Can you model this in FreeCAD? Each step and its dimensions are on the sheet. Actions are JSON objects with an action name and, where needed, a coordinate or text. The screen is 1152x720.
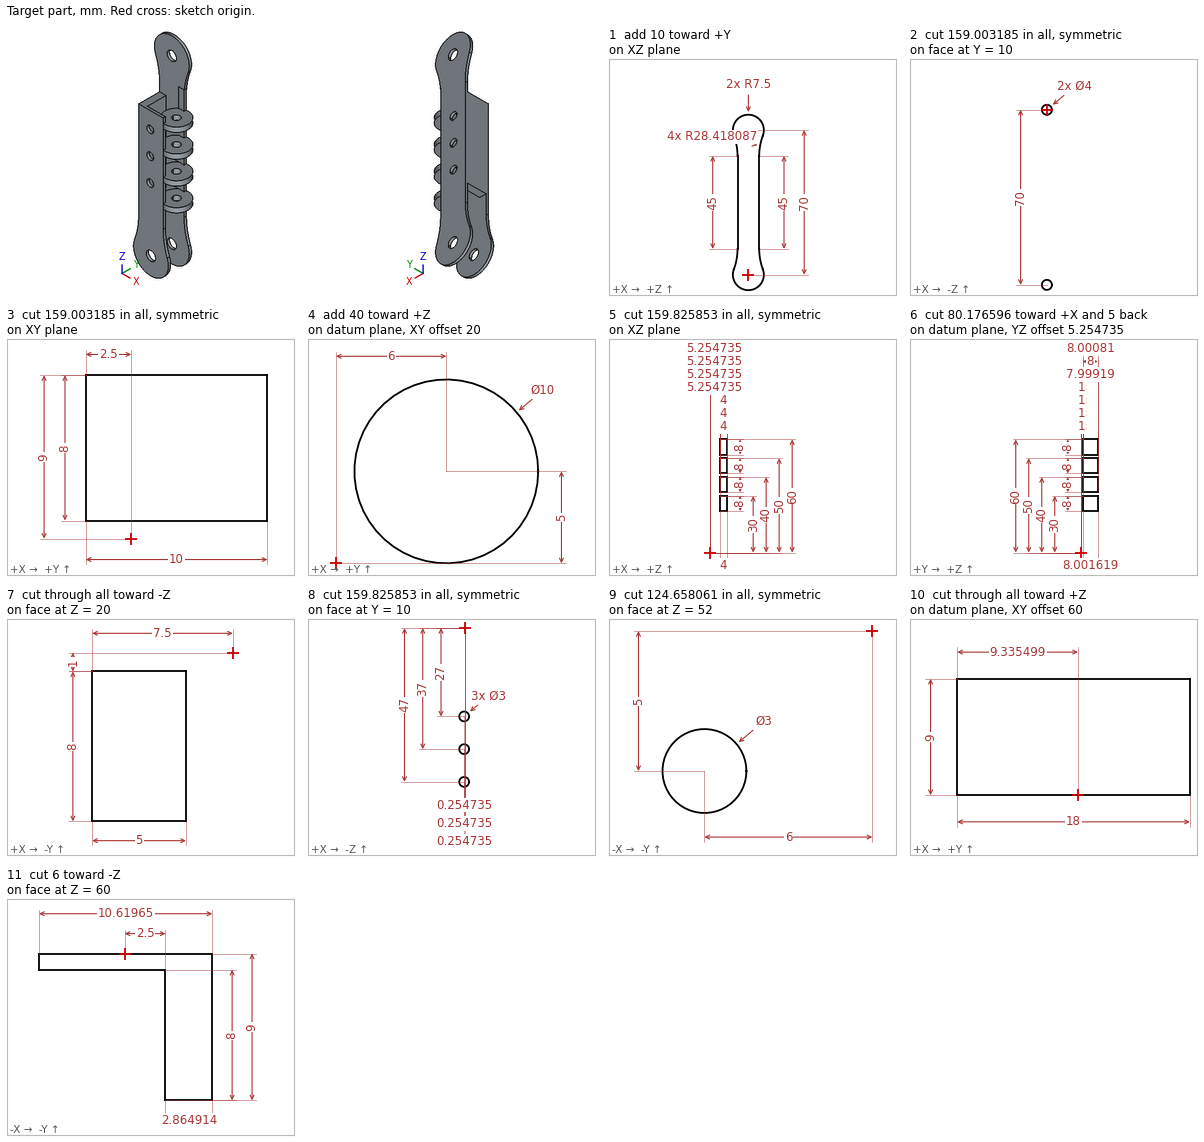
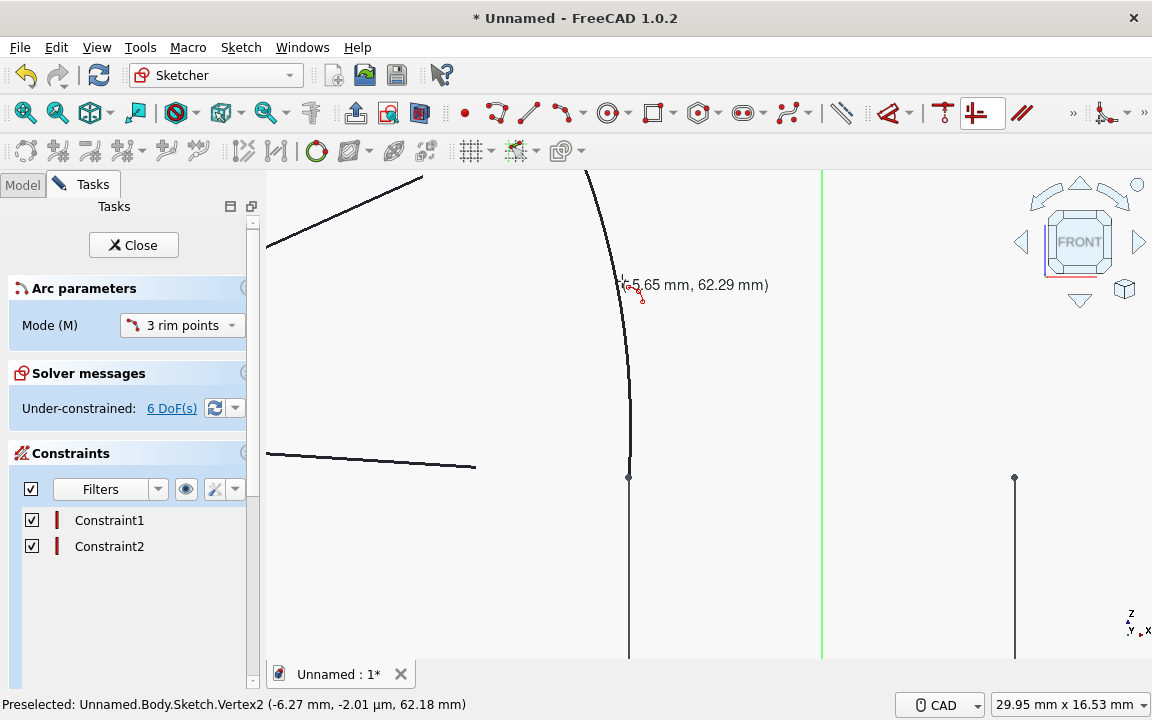
{"action": "left_click", "coordinate": [616, 281]}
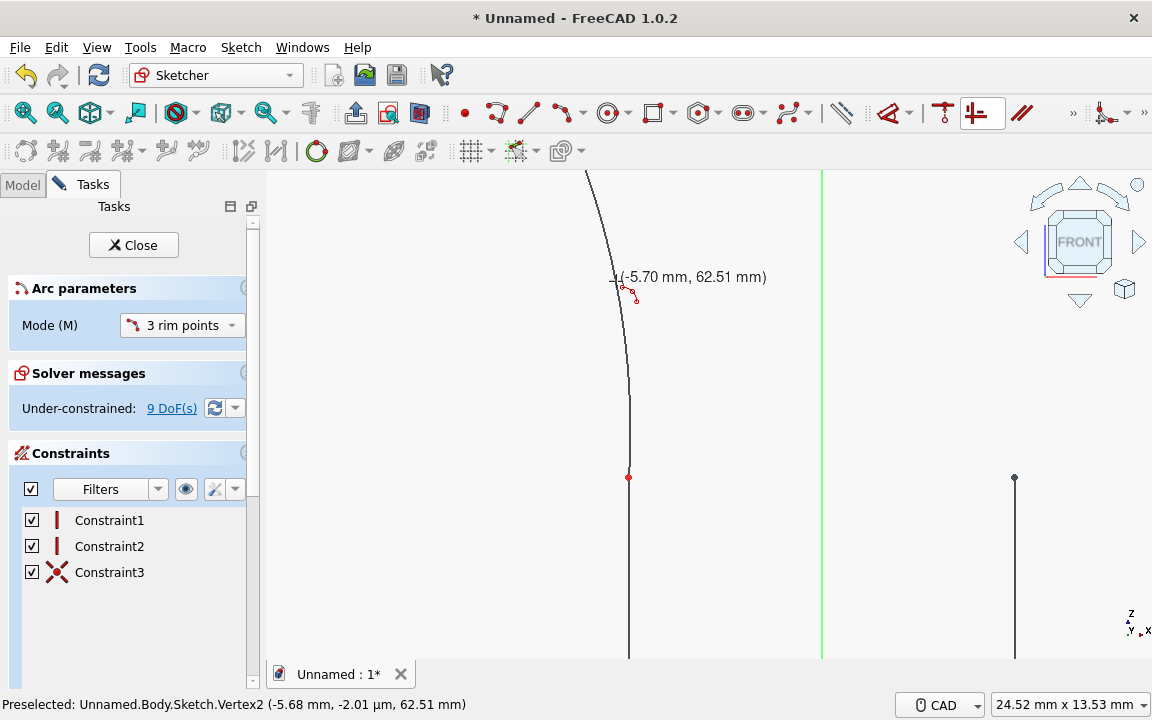
{"action": "scroll", "coordinate": [622, 329], "scroll_direction": "down", "scroll_amount": 12}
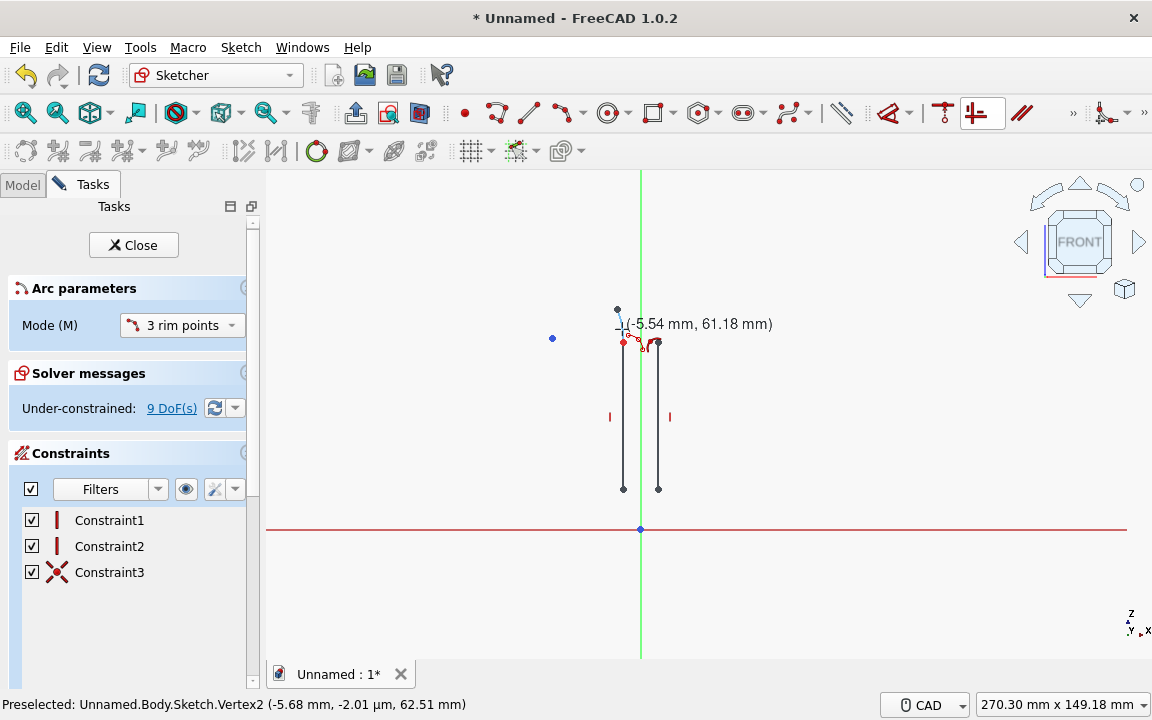
{"action": "left_click", "coordinate": [617, 310]}
{"action": "left_click", "coordinate": [664, 309]}
{"action": "left_click", "coordinate": [658, 283]}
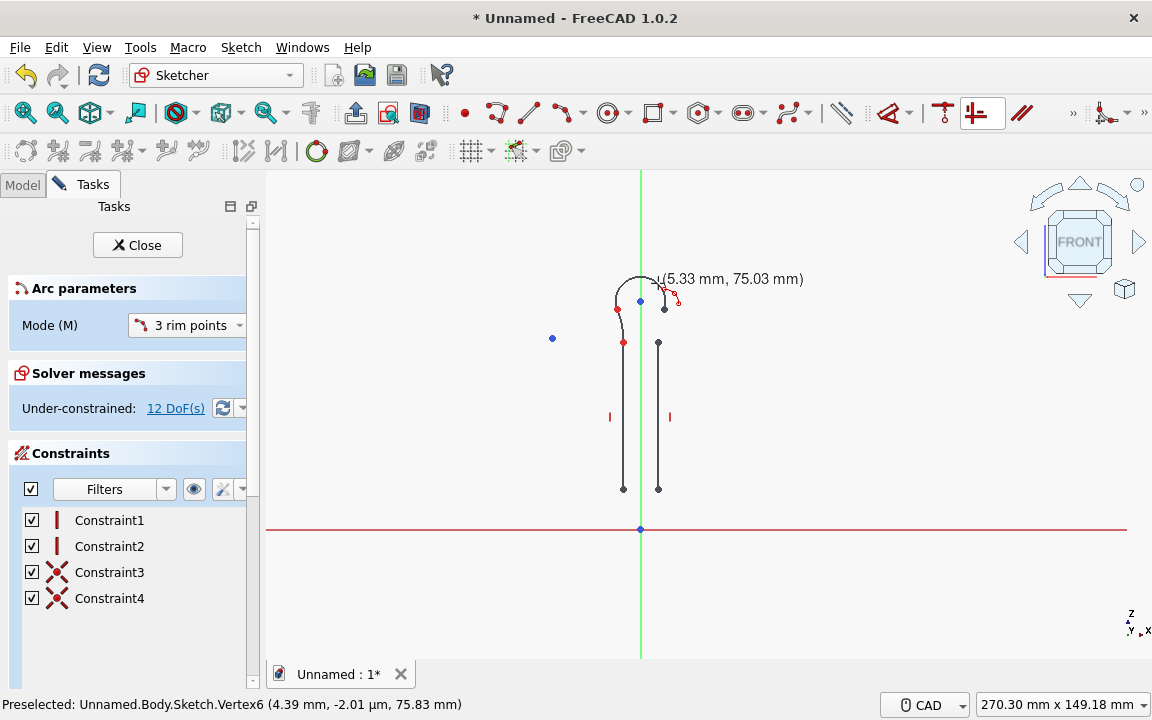
{"action": "left_click", "coordinate": [664, 310]}
{"action": "left_click", "coordinate": [658, 343]}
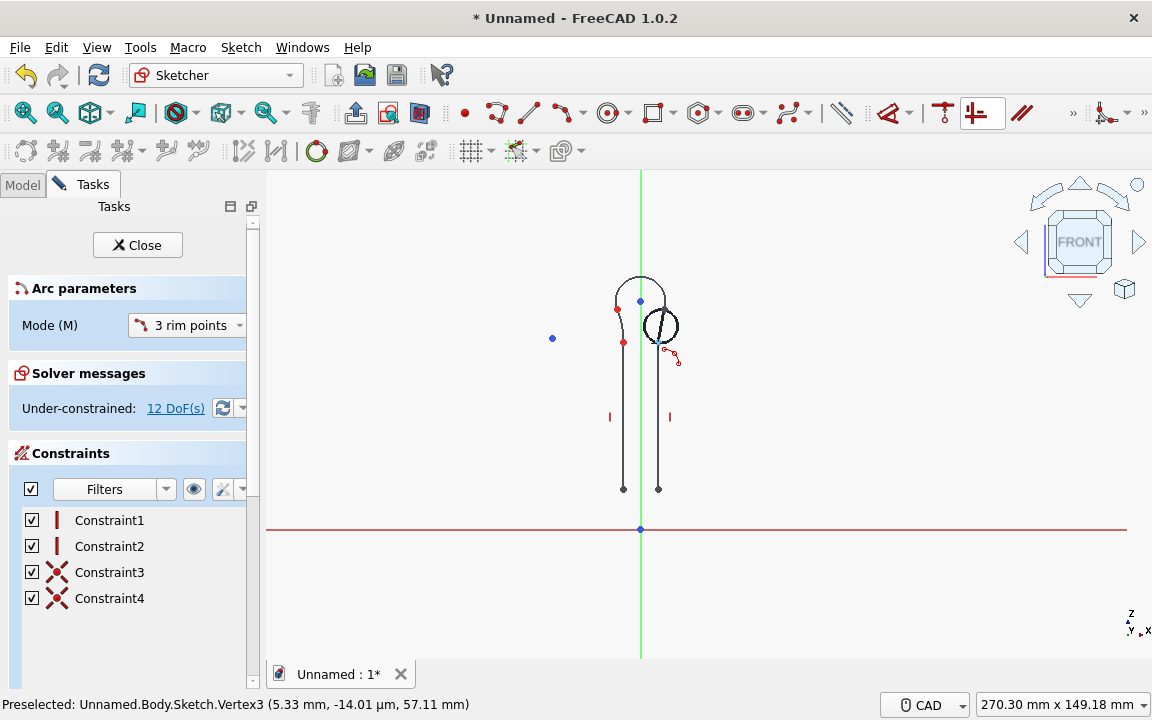
{"action": "scroll", "coordinate": [659, 325], "scroll_direction": "up", "scroll_amount": 12}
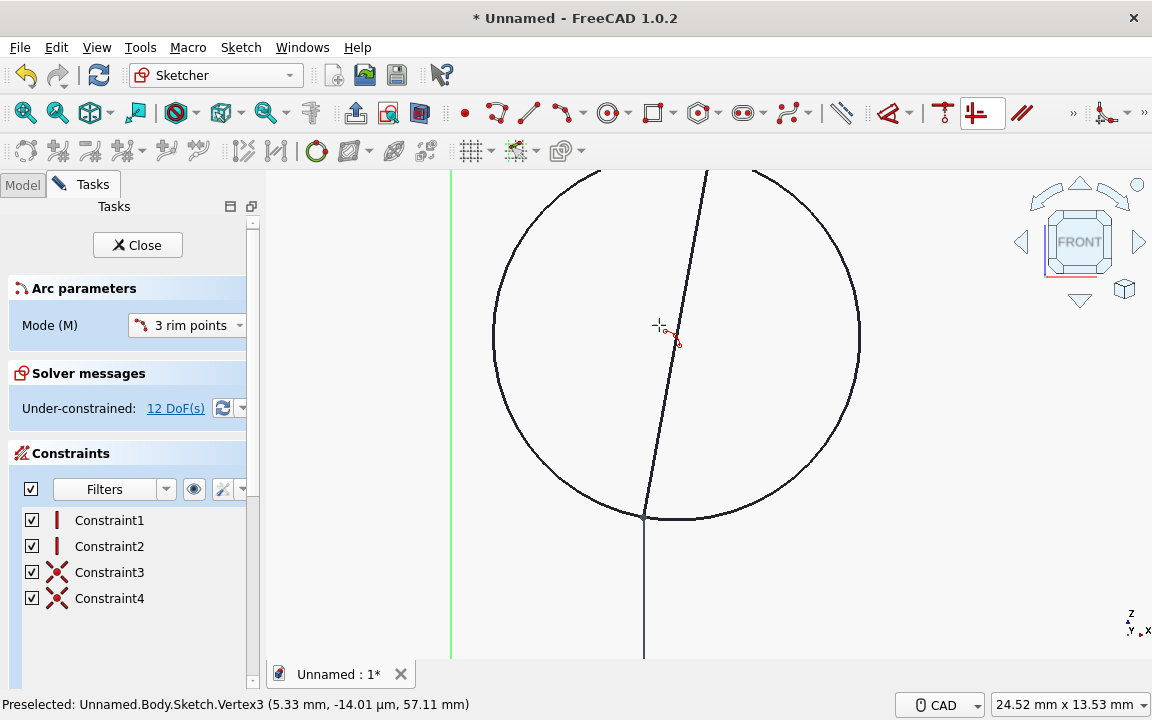
{"action": "left_click", "coordinate": [657, 322]}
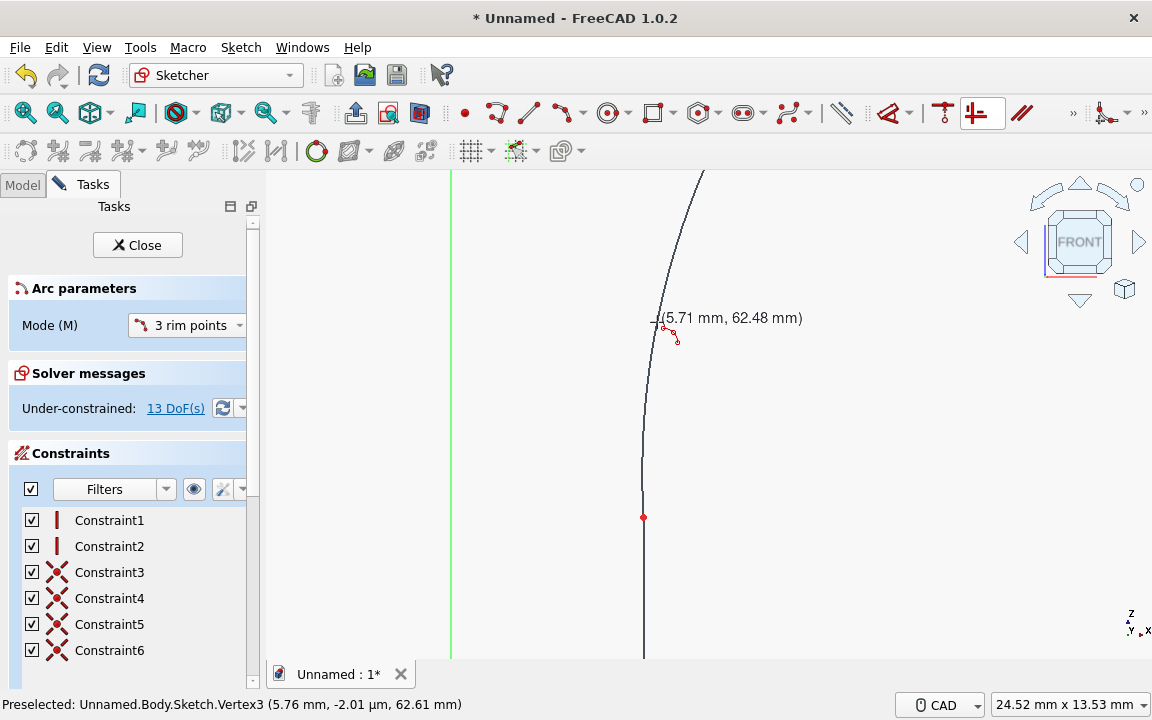
{"action": "scroll", "coordinate": [659, 325], "scroll_direction": "down", "scroll_amount": 12}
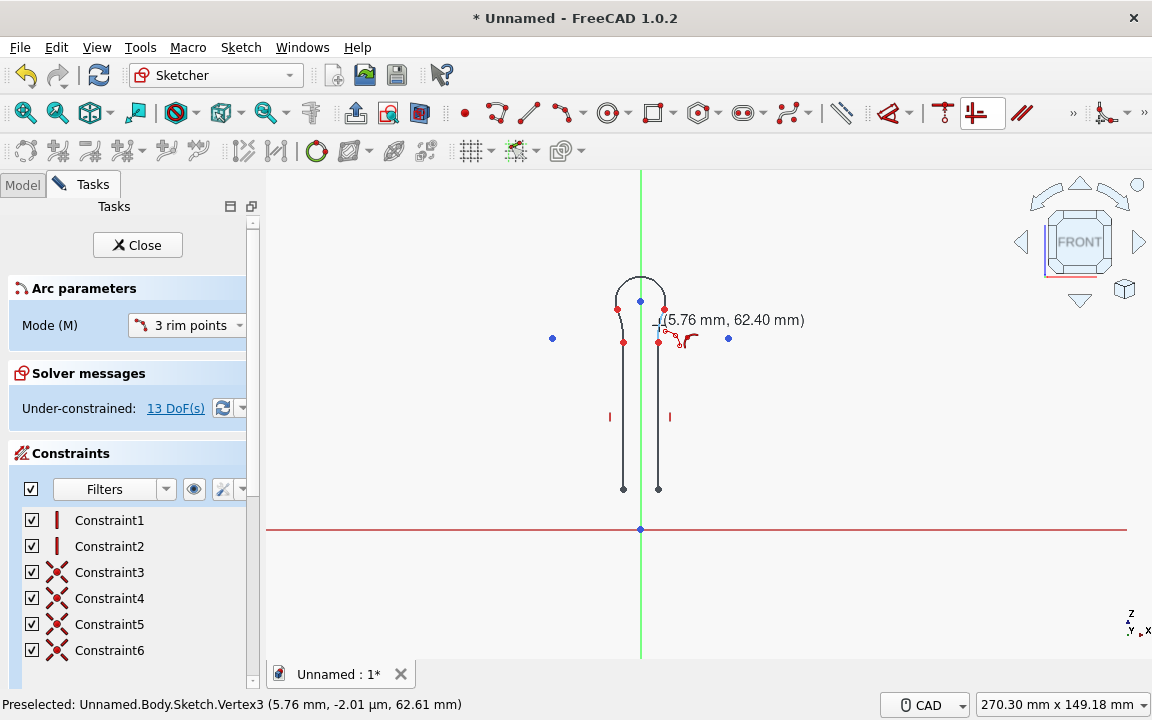
{"action": "left_click", "coordinate": [658, 490]}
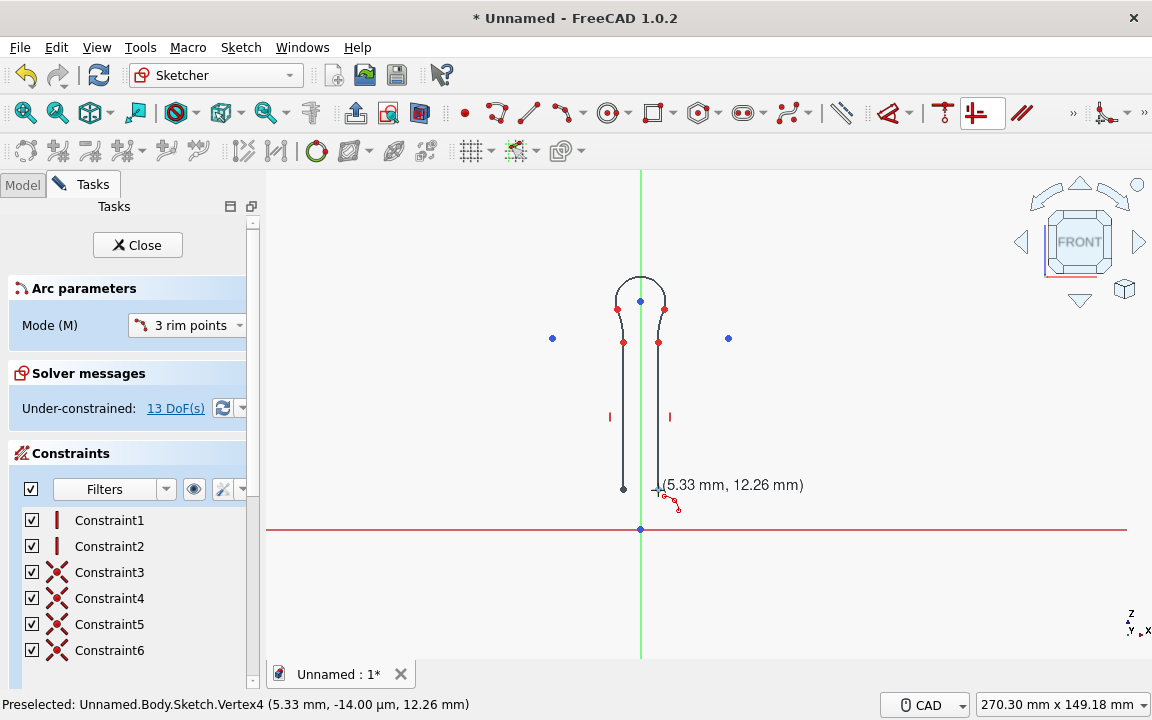
{"action": "scroll", "coordinate": [664, 521], "scroll_direction": "up", "scroll_amount": 4}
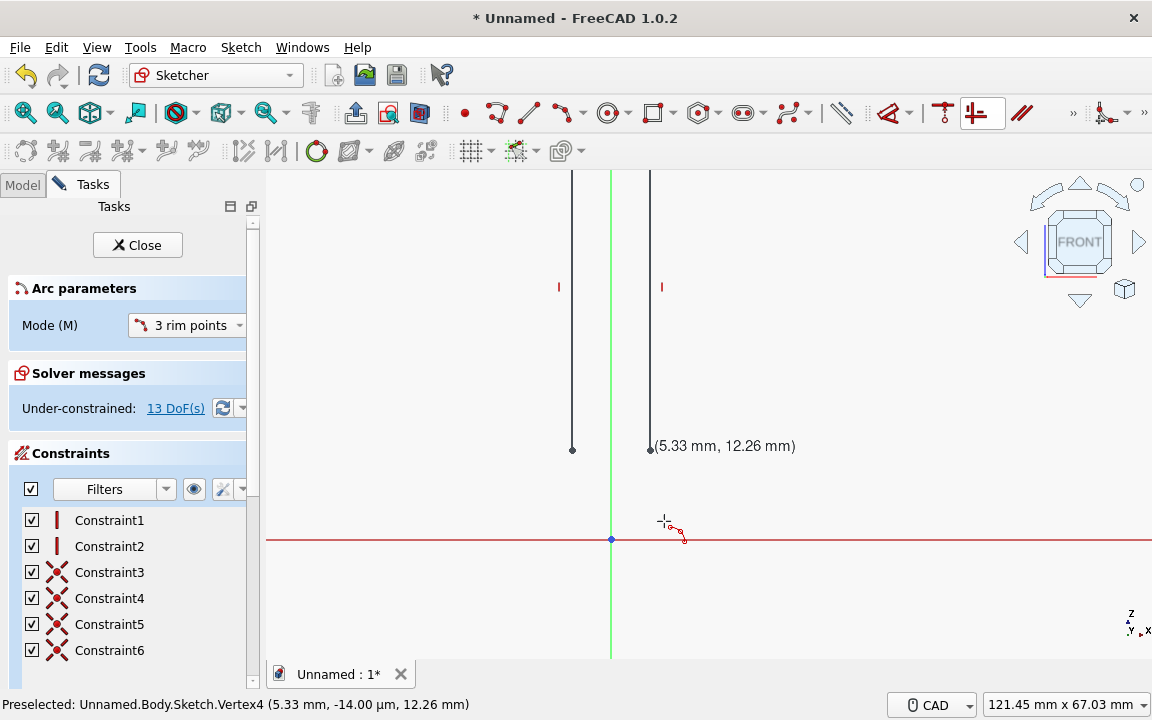
{"action": "left_click", "coordinate": [662, 521]}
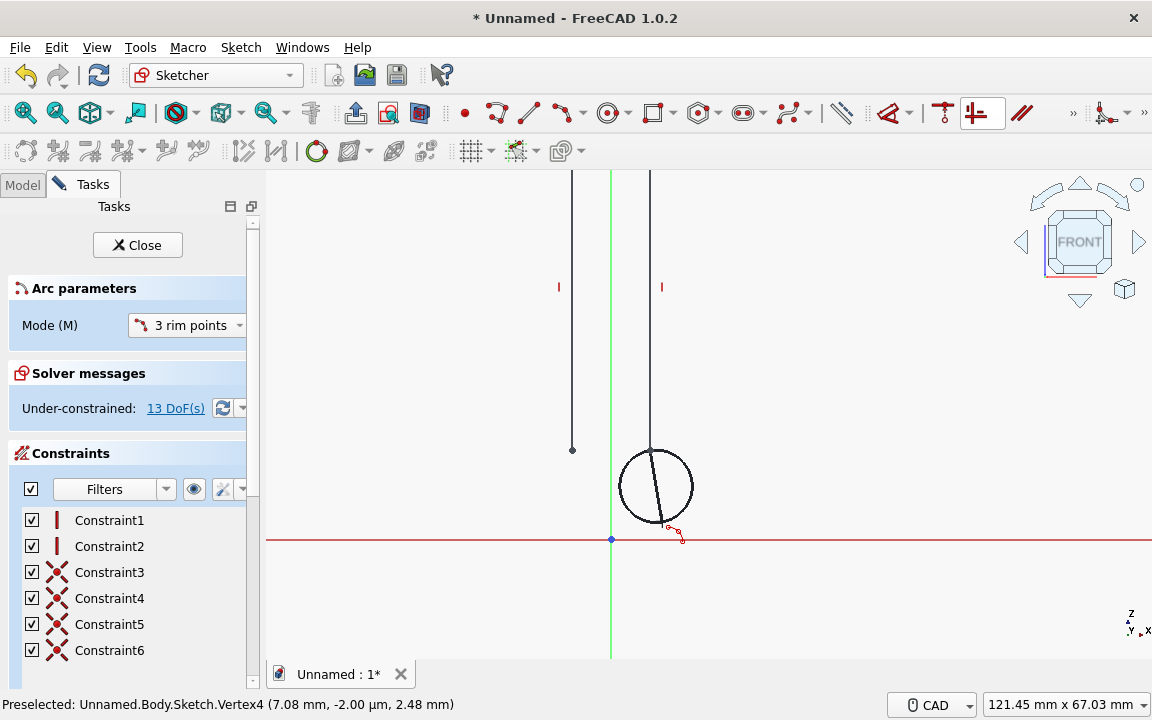
{"action": "scroll", "coordinate": [653, 485], "scroll_direction": "up", "scroll_amount": 8}